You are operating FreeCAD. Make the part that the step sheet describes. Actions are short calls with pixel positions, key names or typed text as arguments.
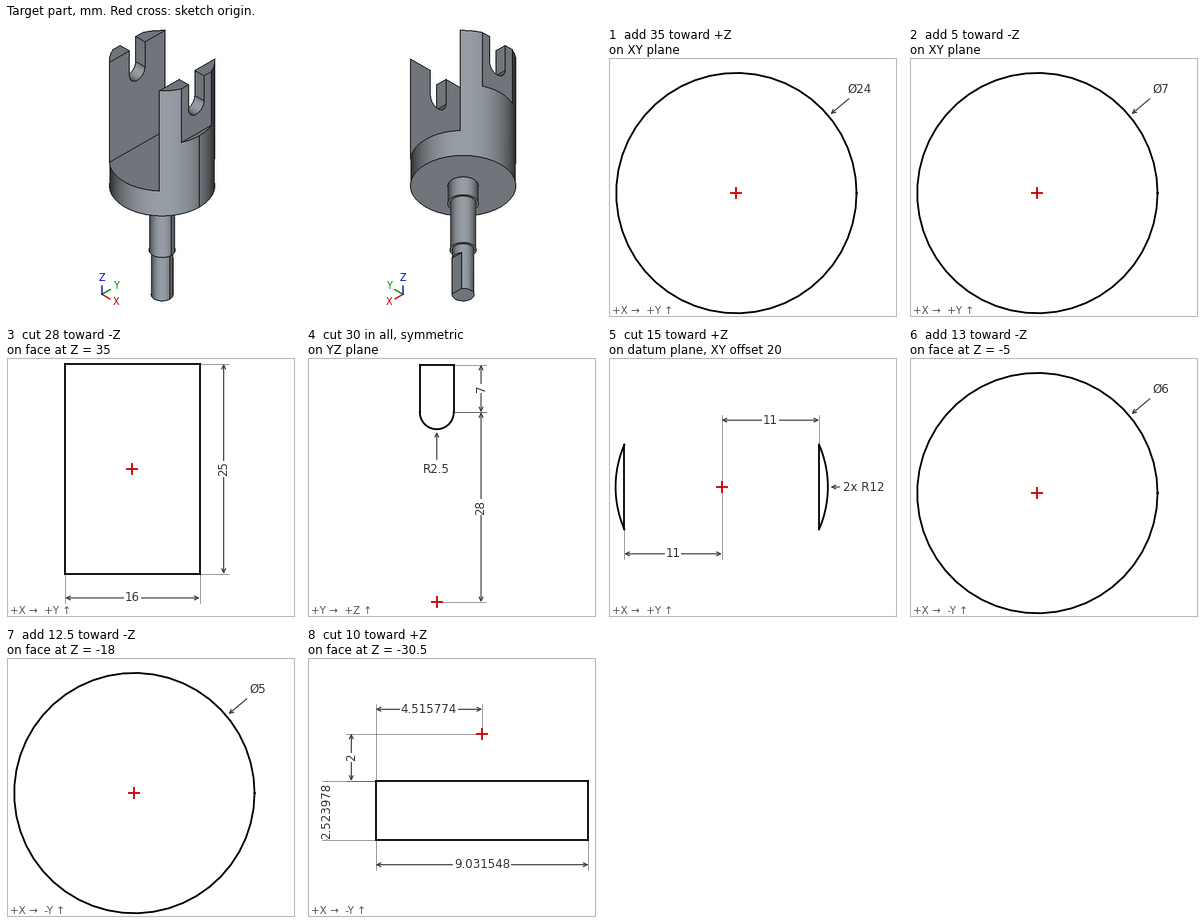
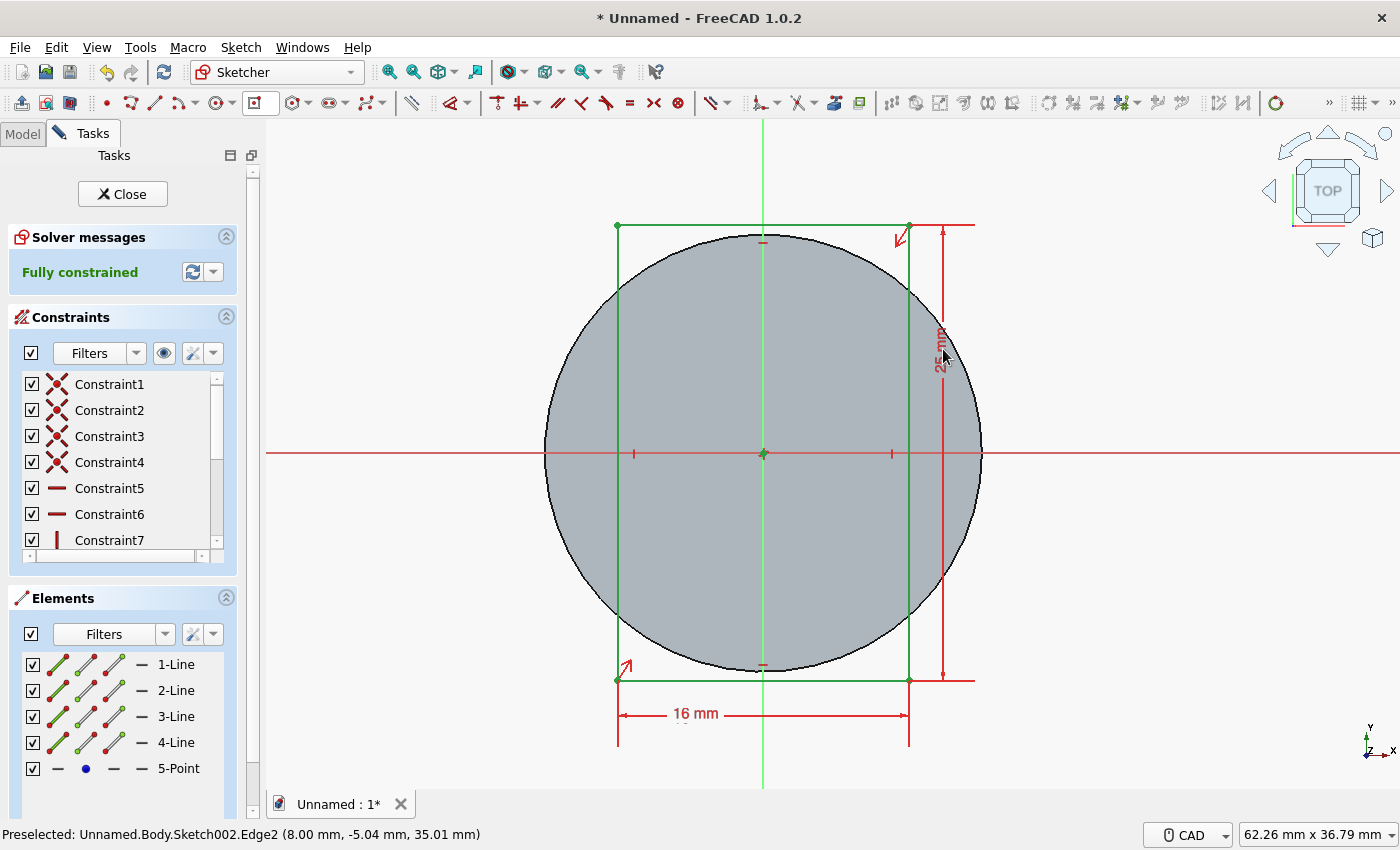
click(123, 194)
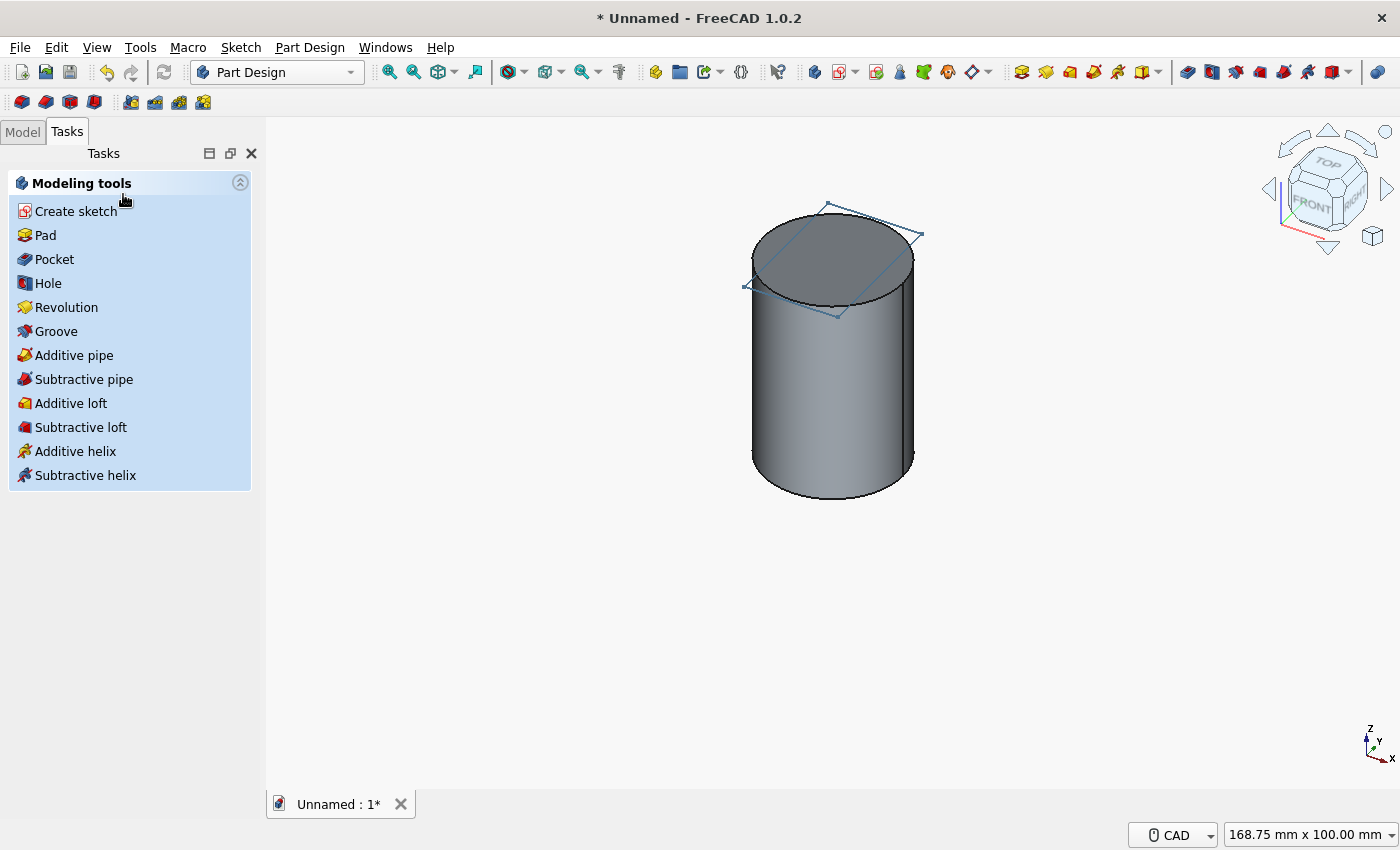
click(1188, 72)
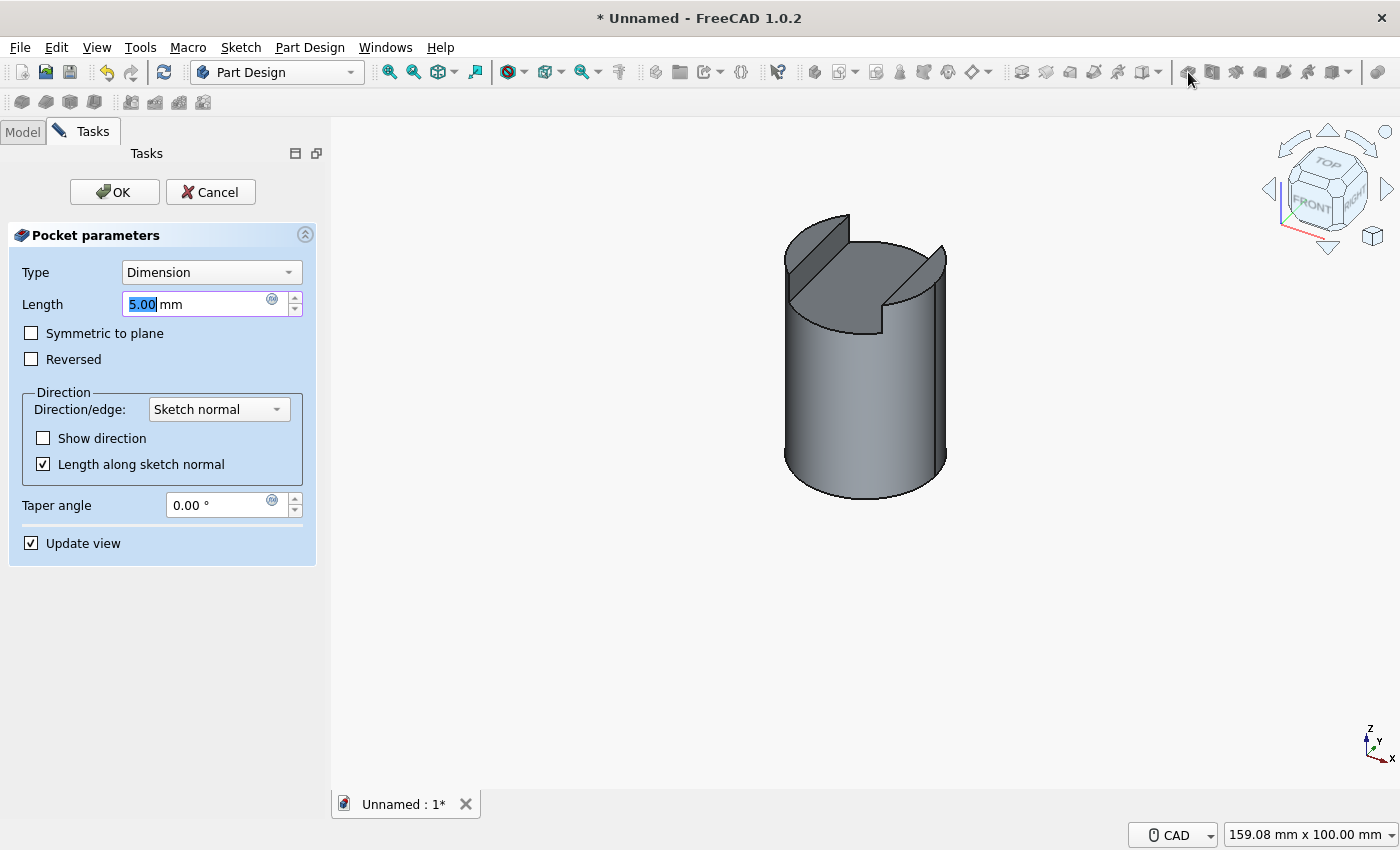
text(28)
key(Tab)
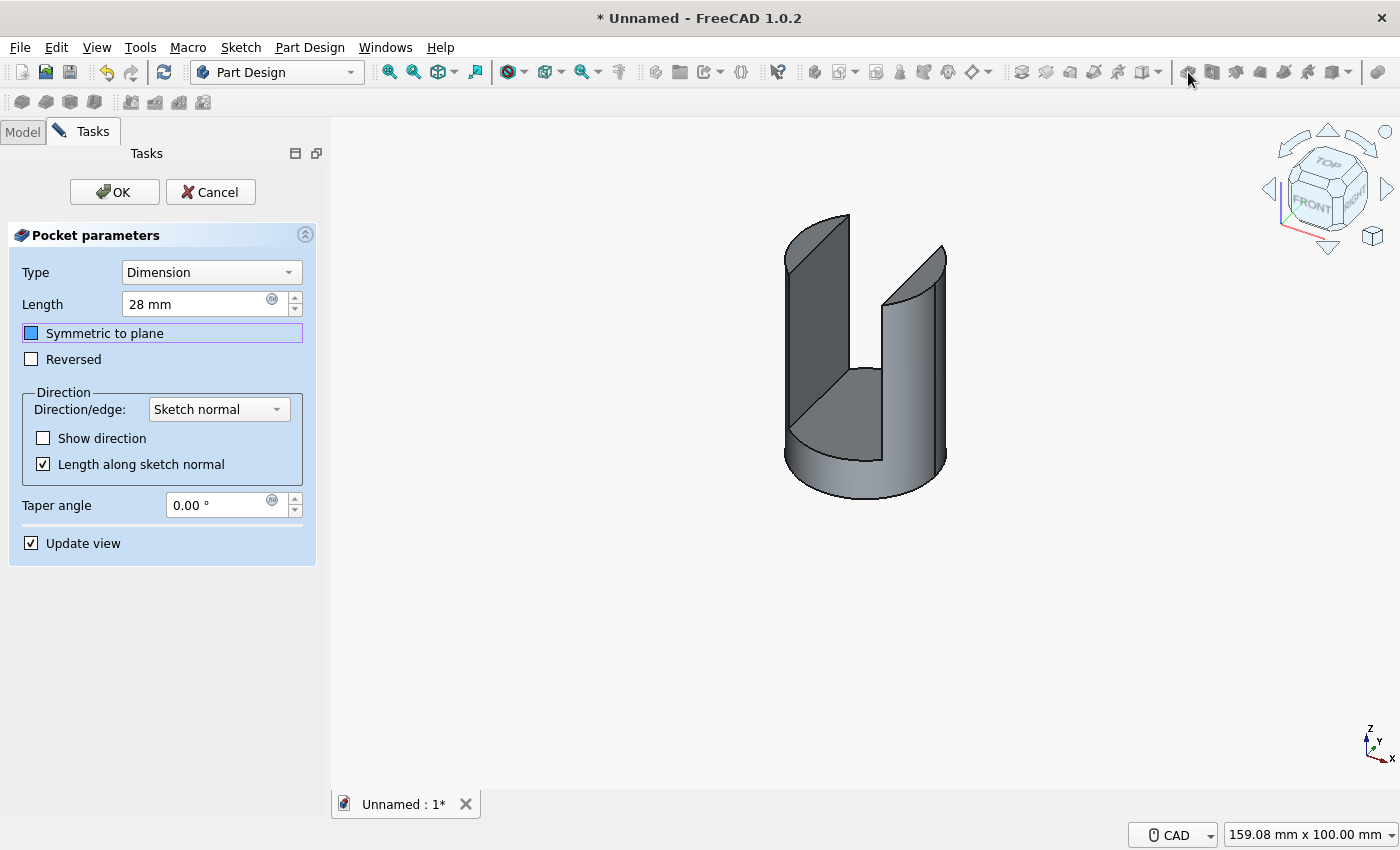
click(115, 192)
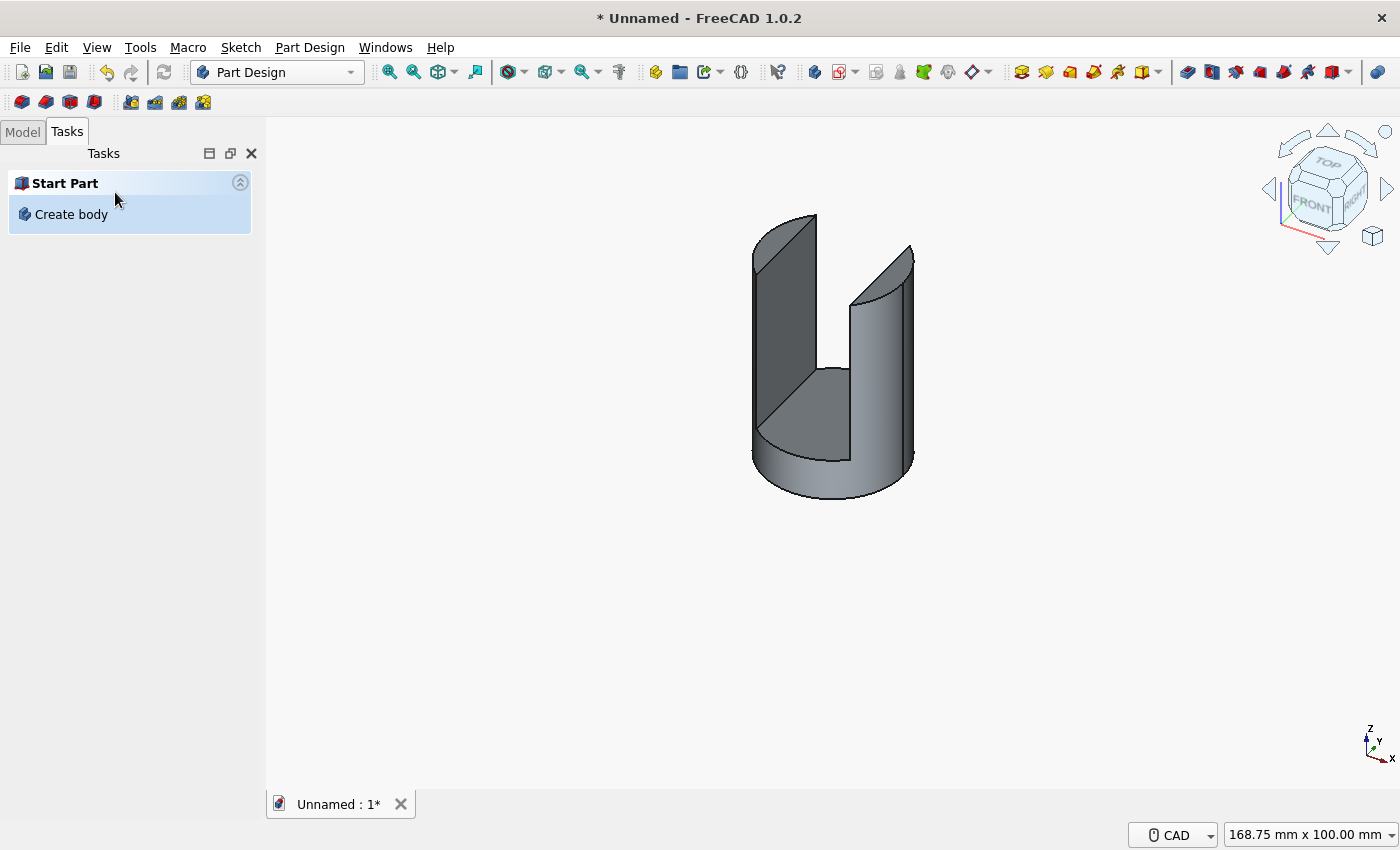
click(840, 72)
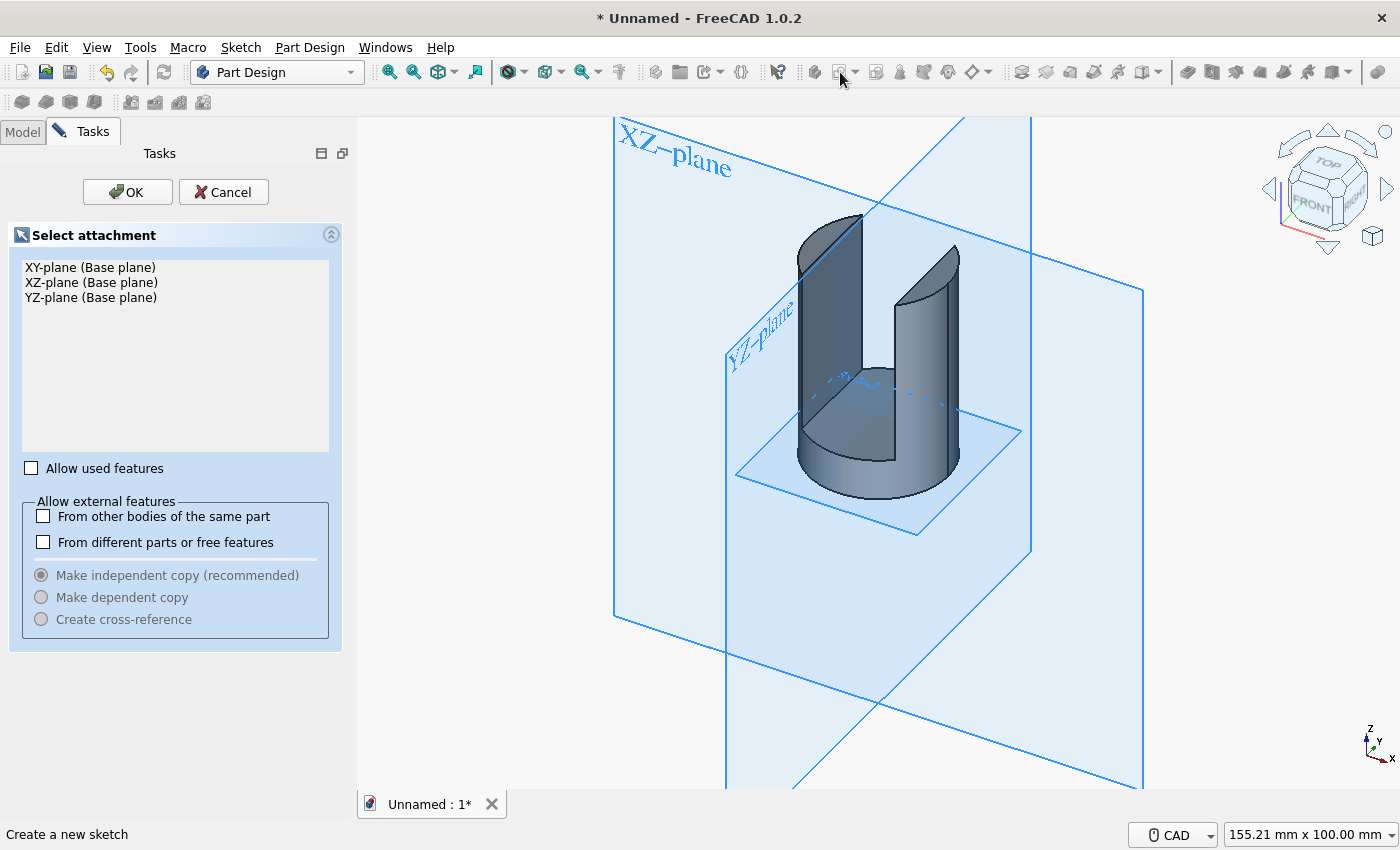
click(82, 298)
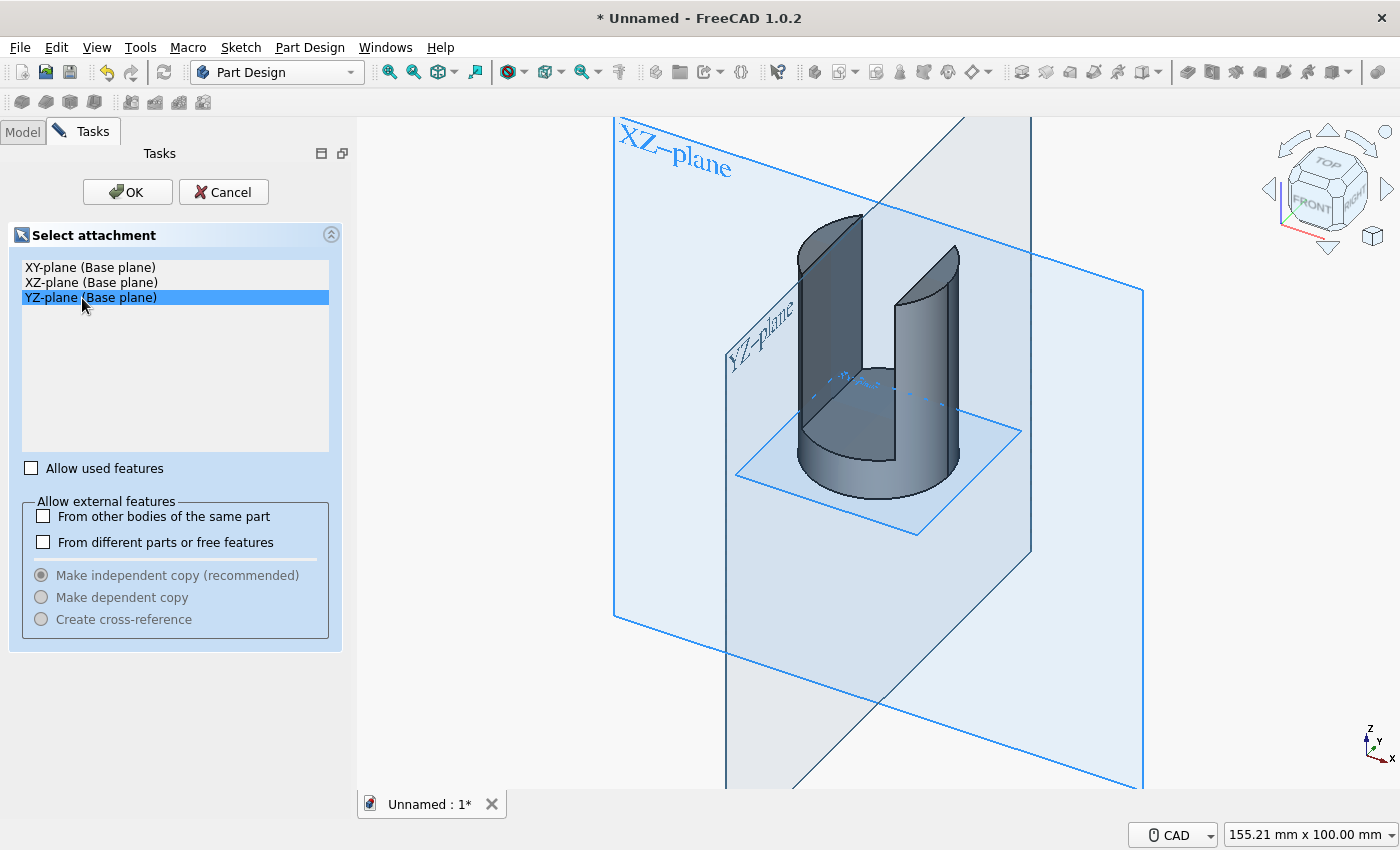
click(128, 192)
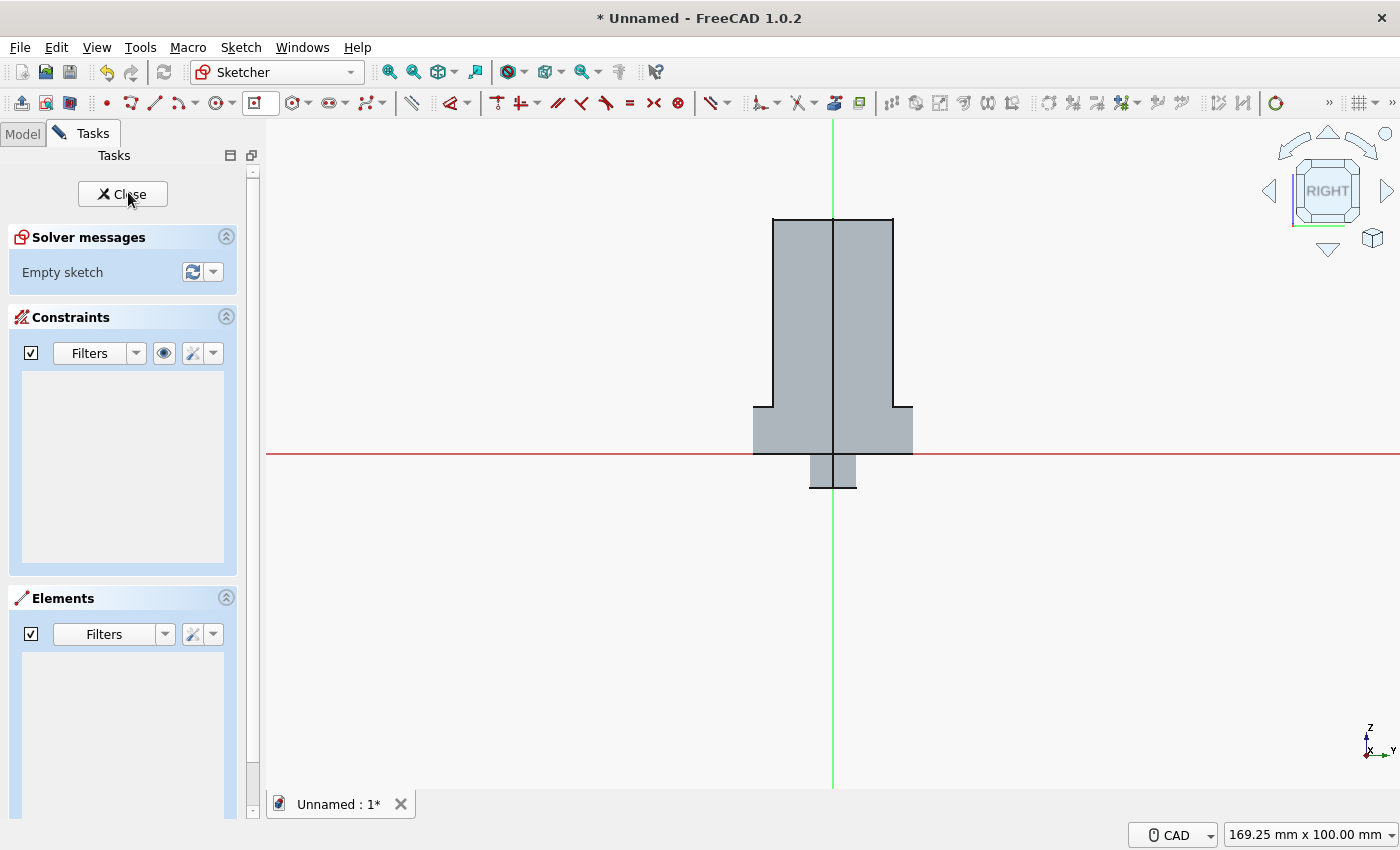
click(70, 104)